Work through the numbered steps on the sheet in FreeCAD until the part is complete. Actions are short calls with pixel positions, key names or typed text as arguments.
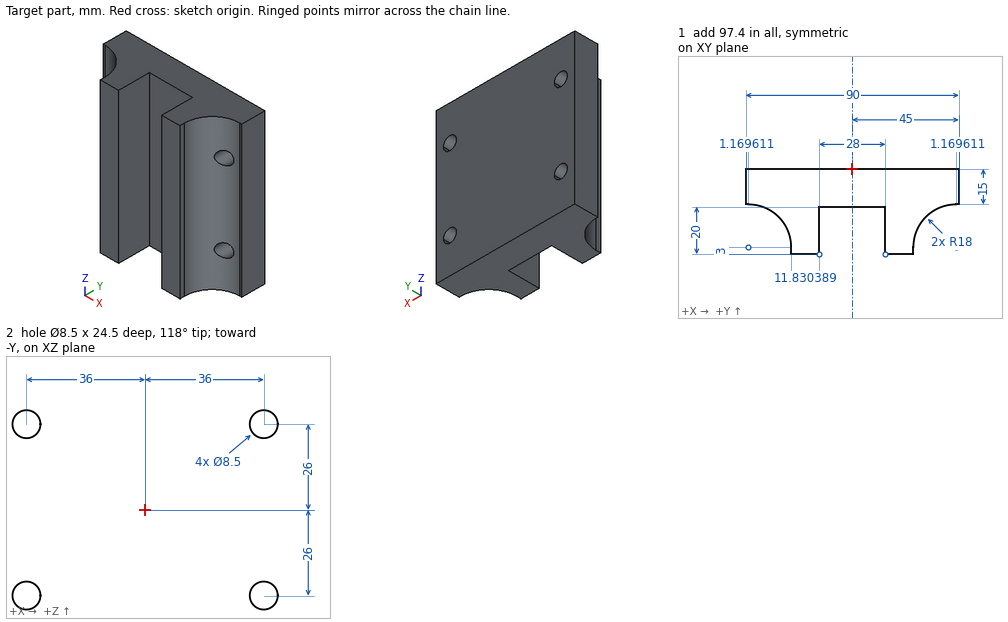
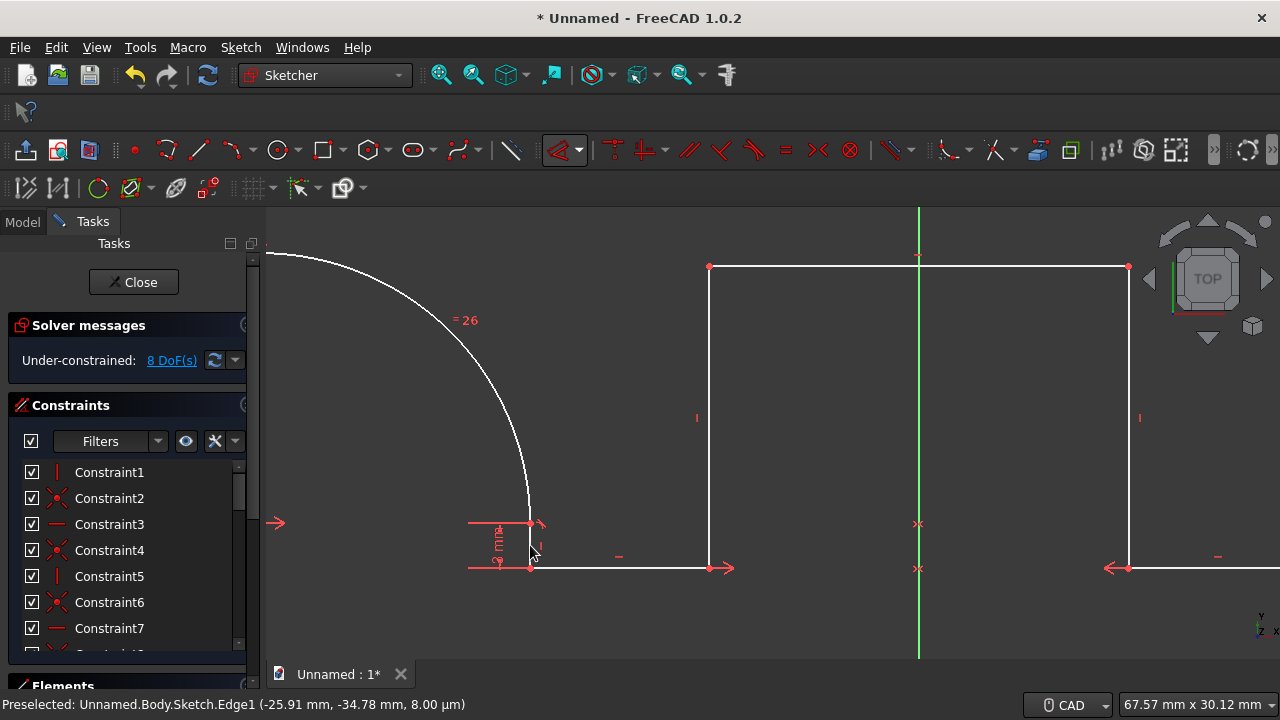
click(709, 478)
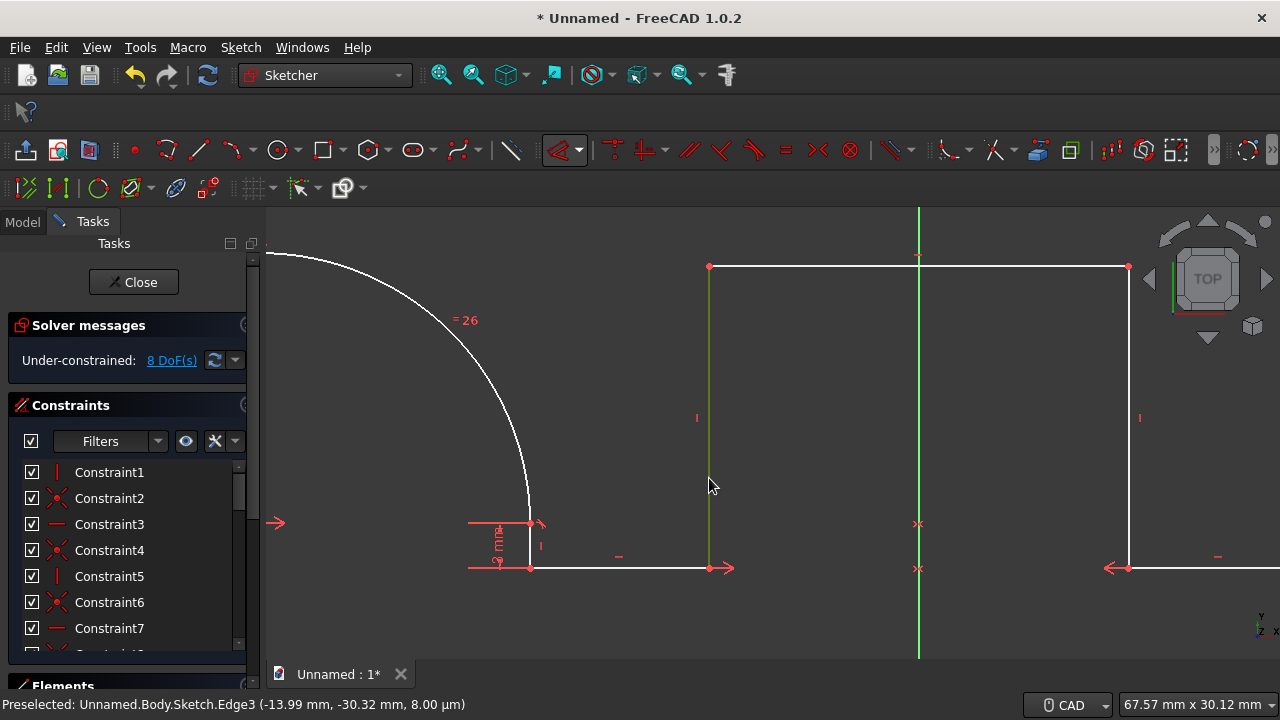
key(i)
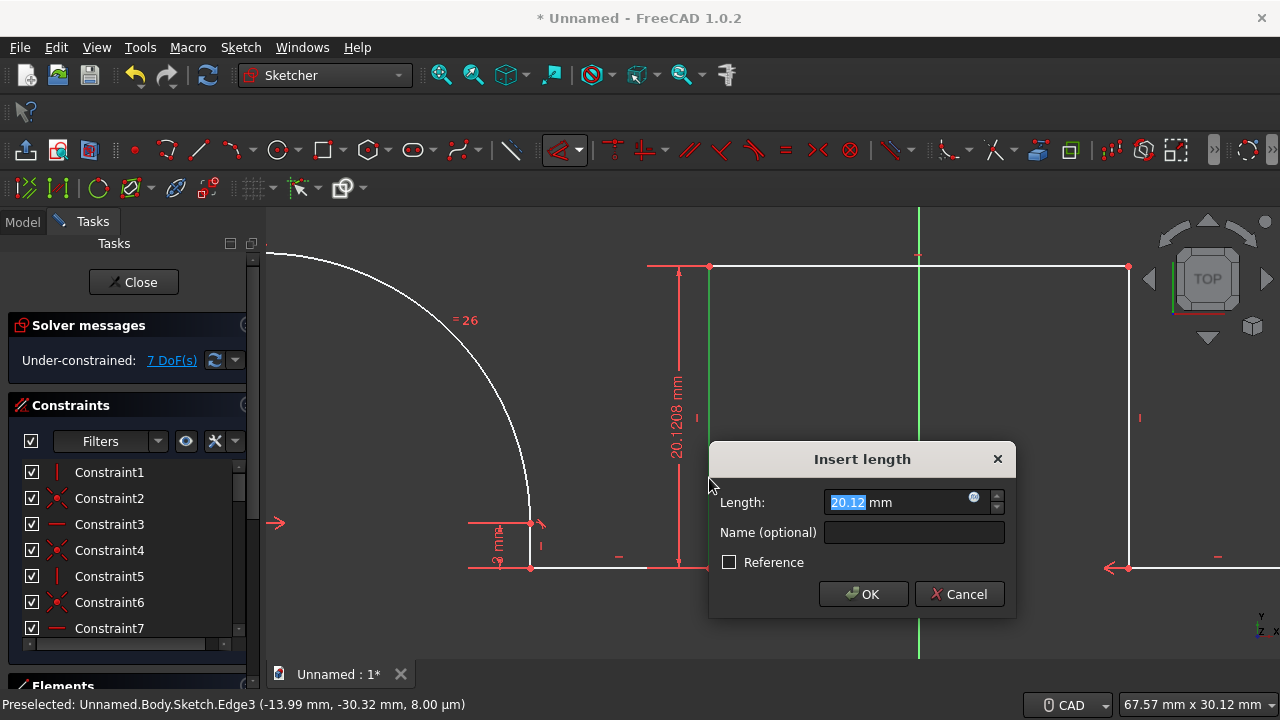
text(20)
key(Return)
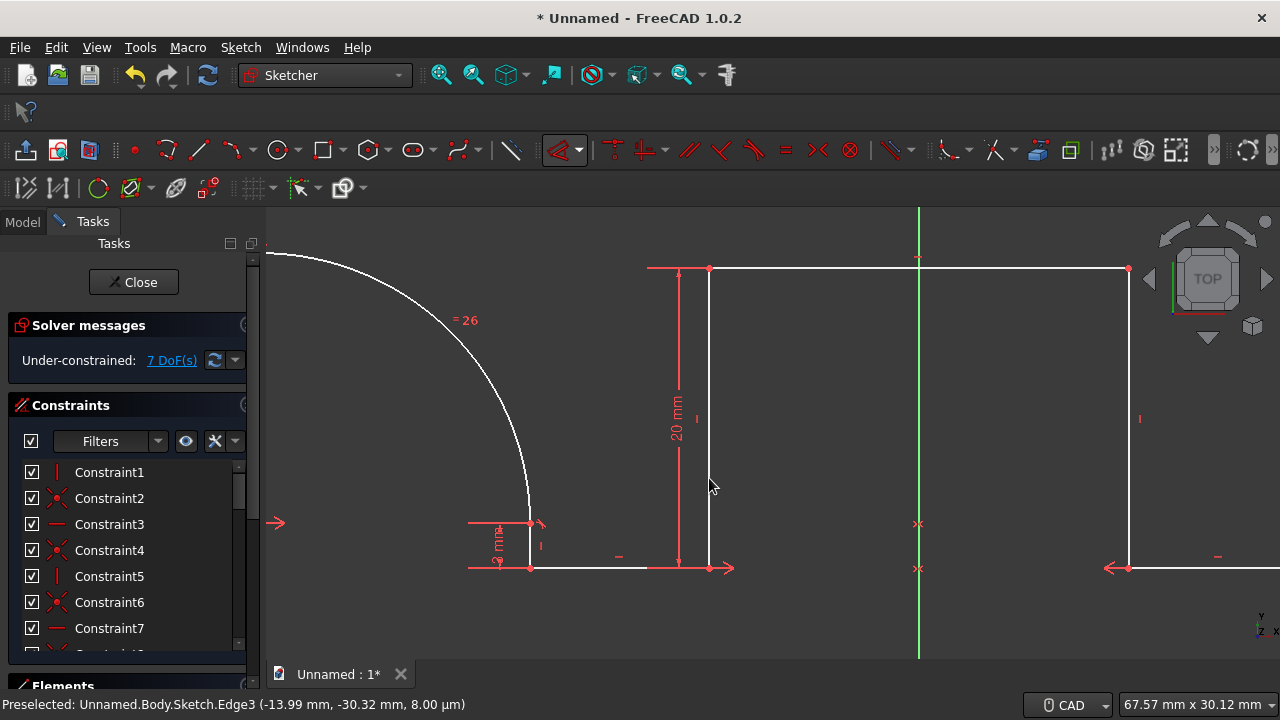
click(835, 268)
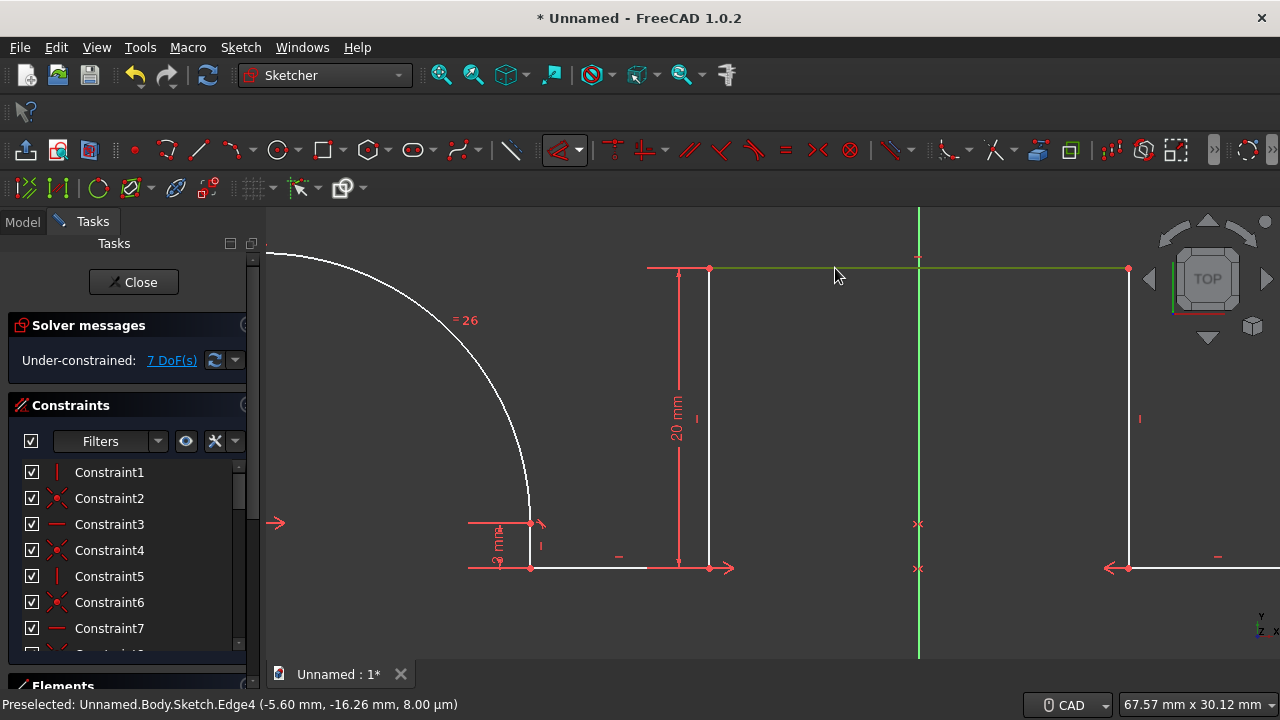
key(l)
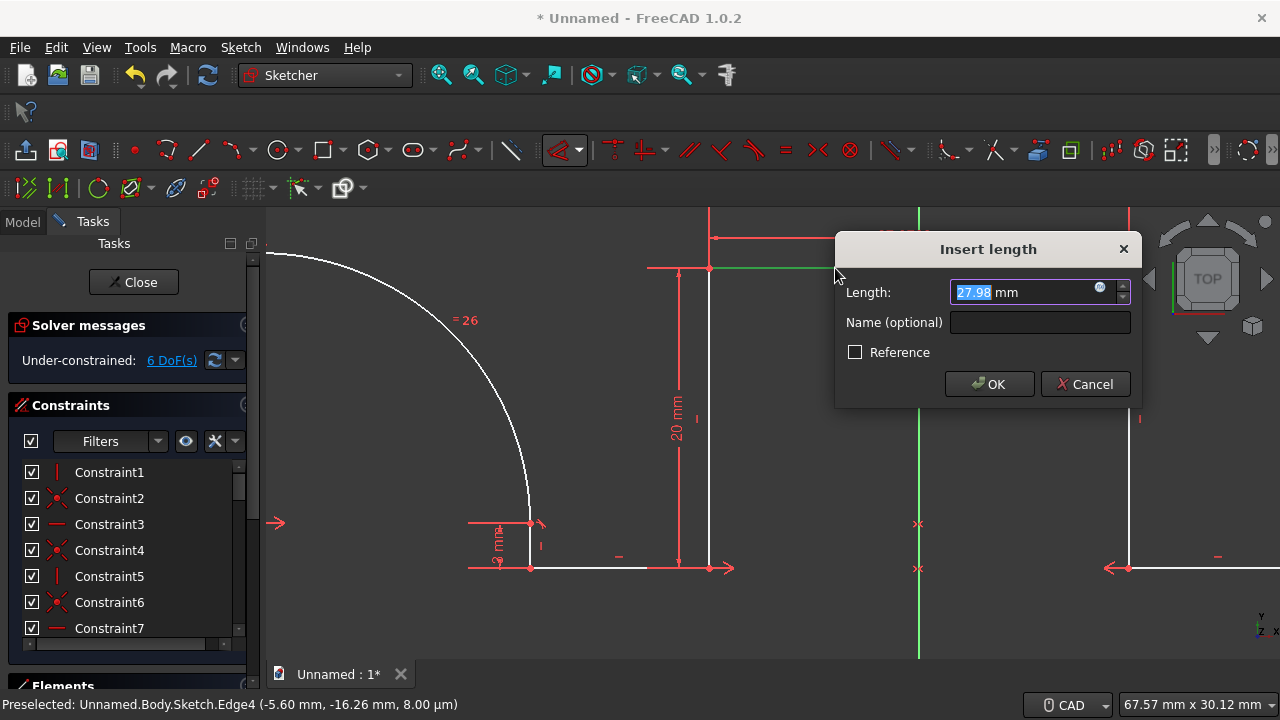
text(28)
key(Return)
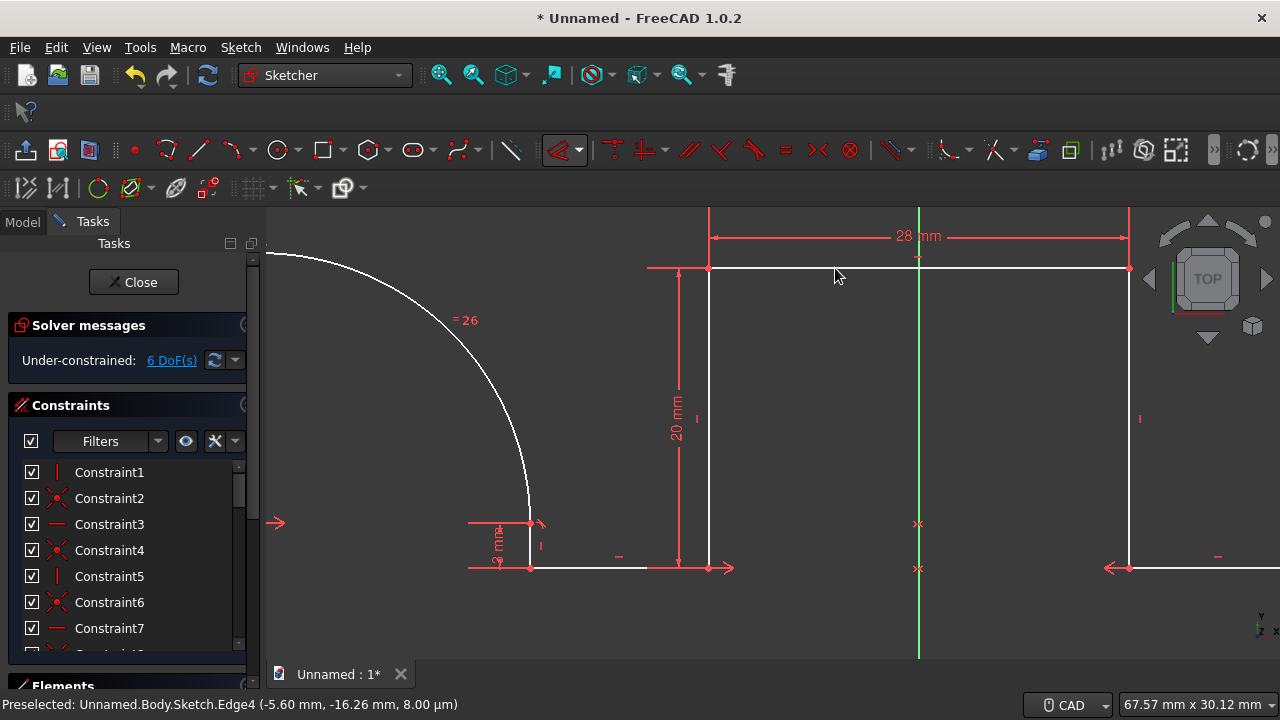
scroll(530, 546, down, 4)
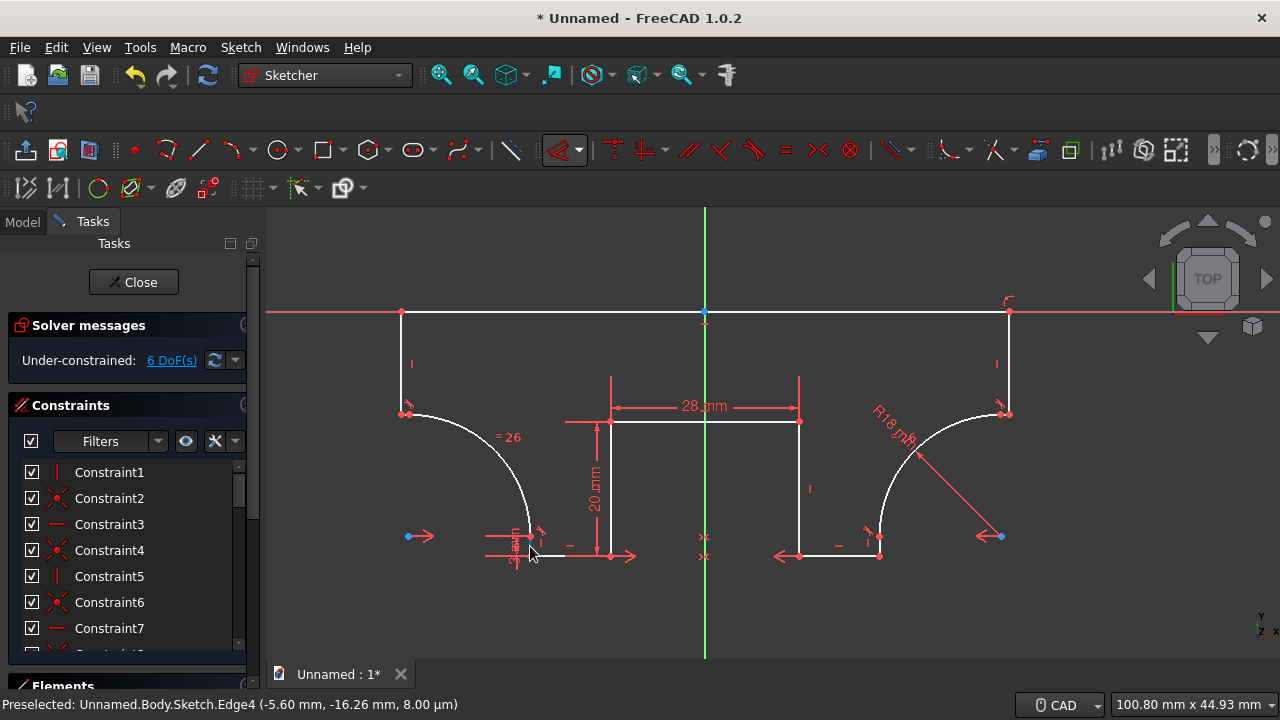
click(1009, 384)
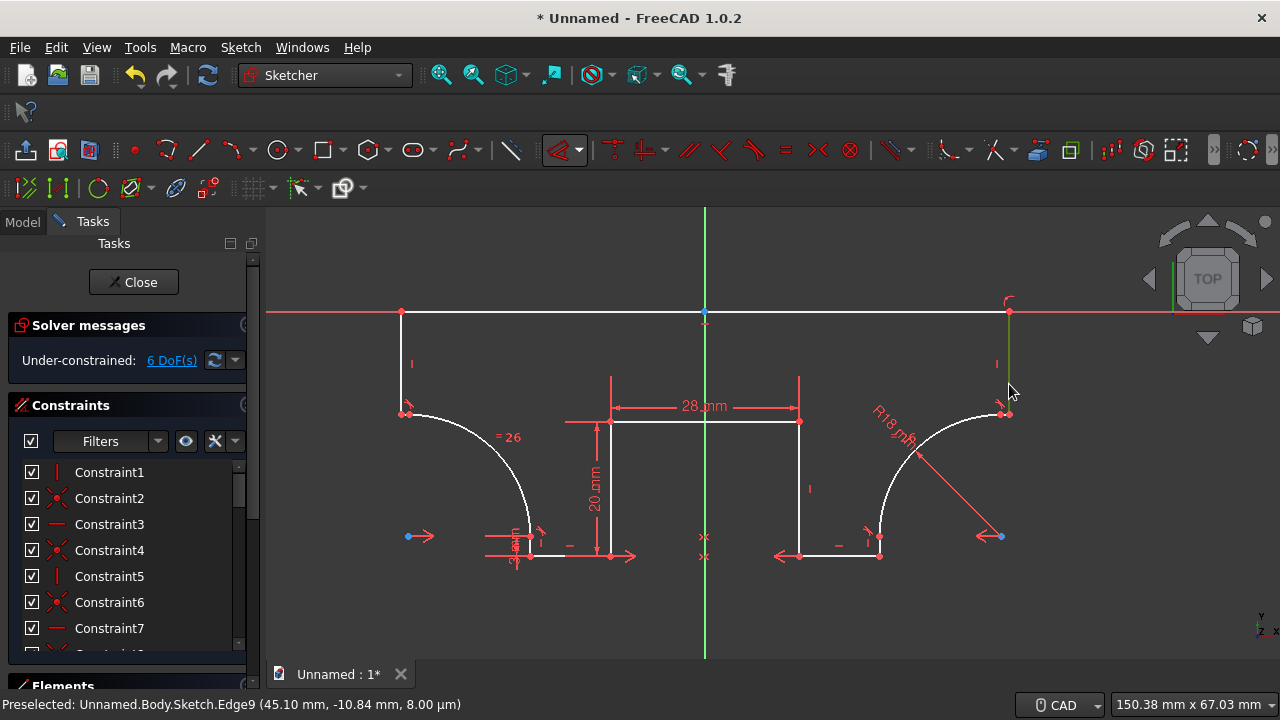
click(582, 150)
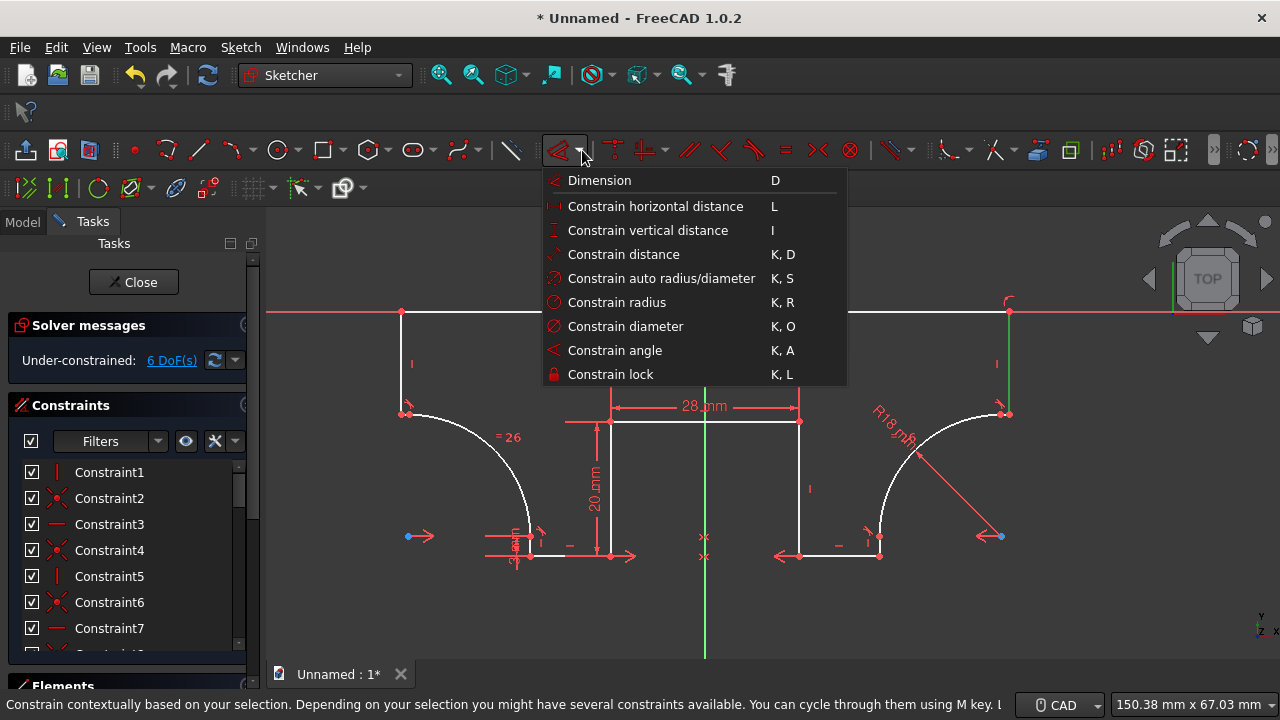
click(695, 230)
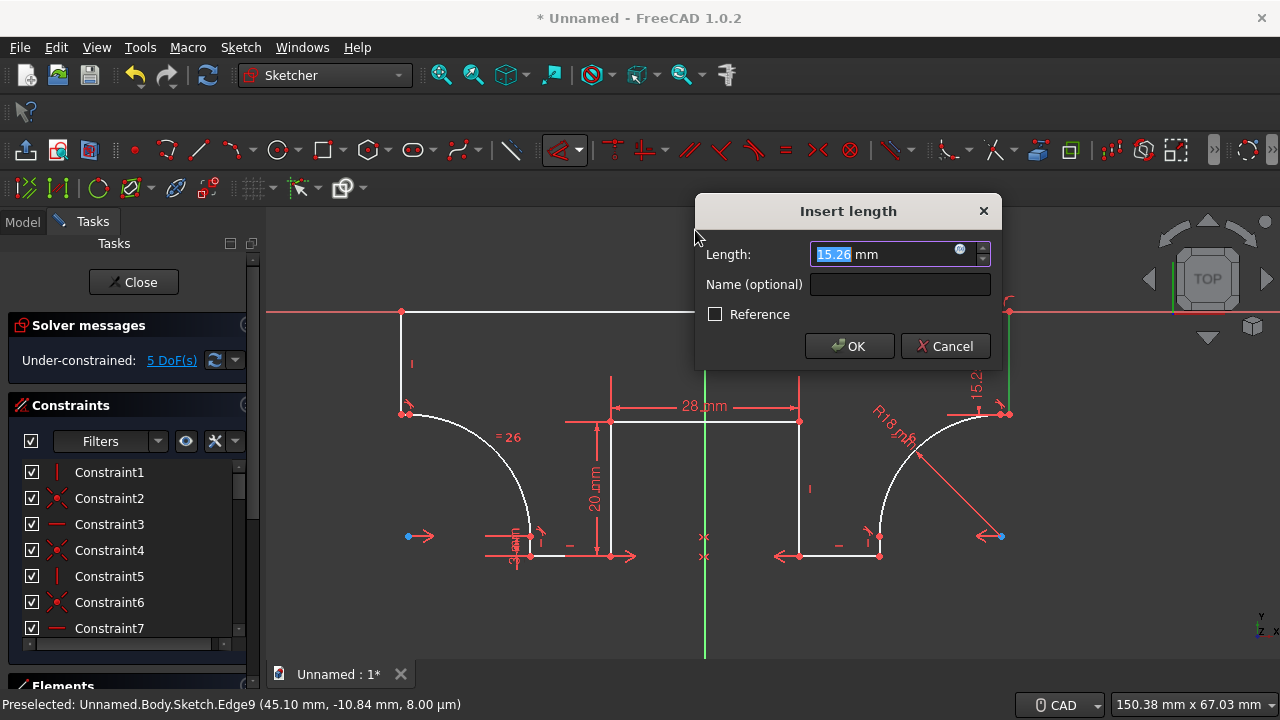
text(15)
key(Return)